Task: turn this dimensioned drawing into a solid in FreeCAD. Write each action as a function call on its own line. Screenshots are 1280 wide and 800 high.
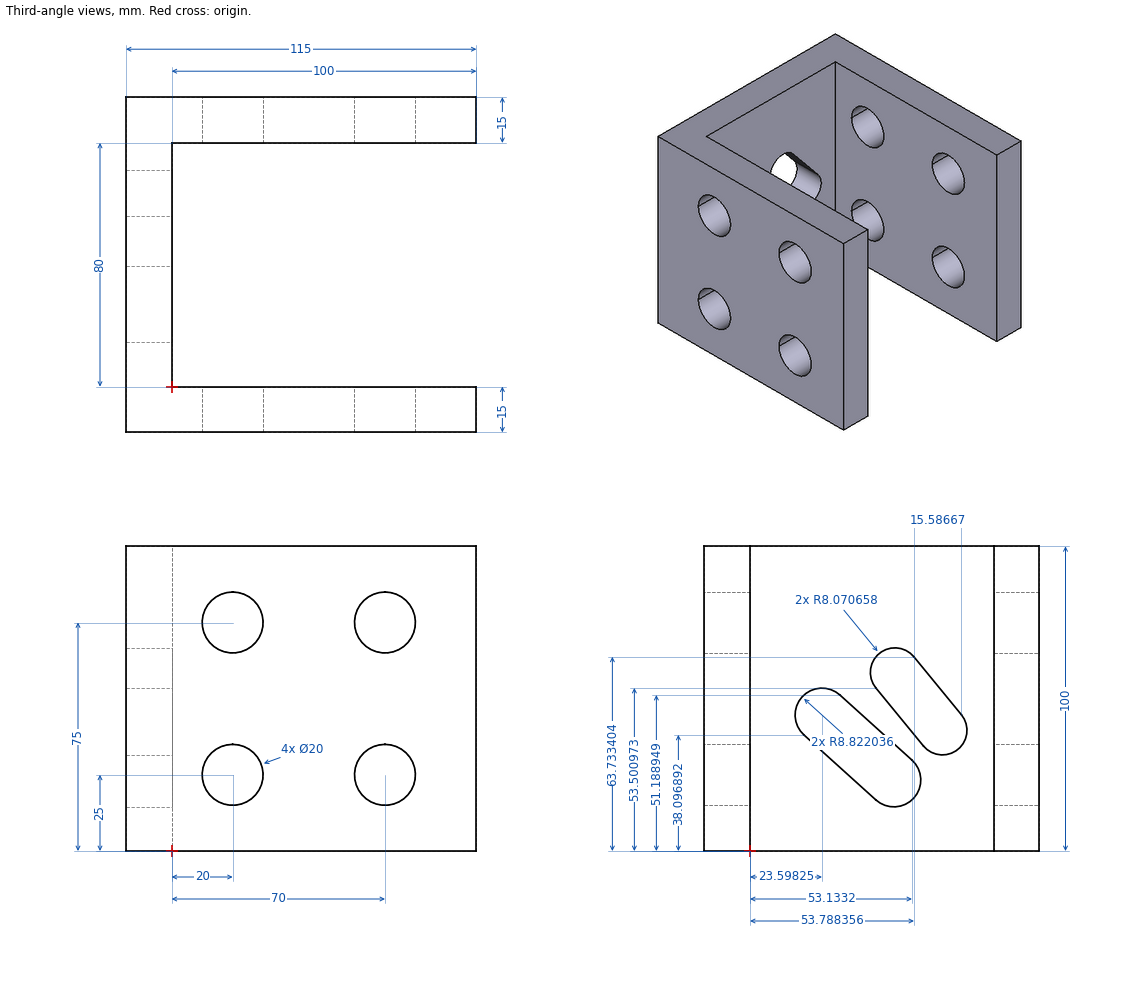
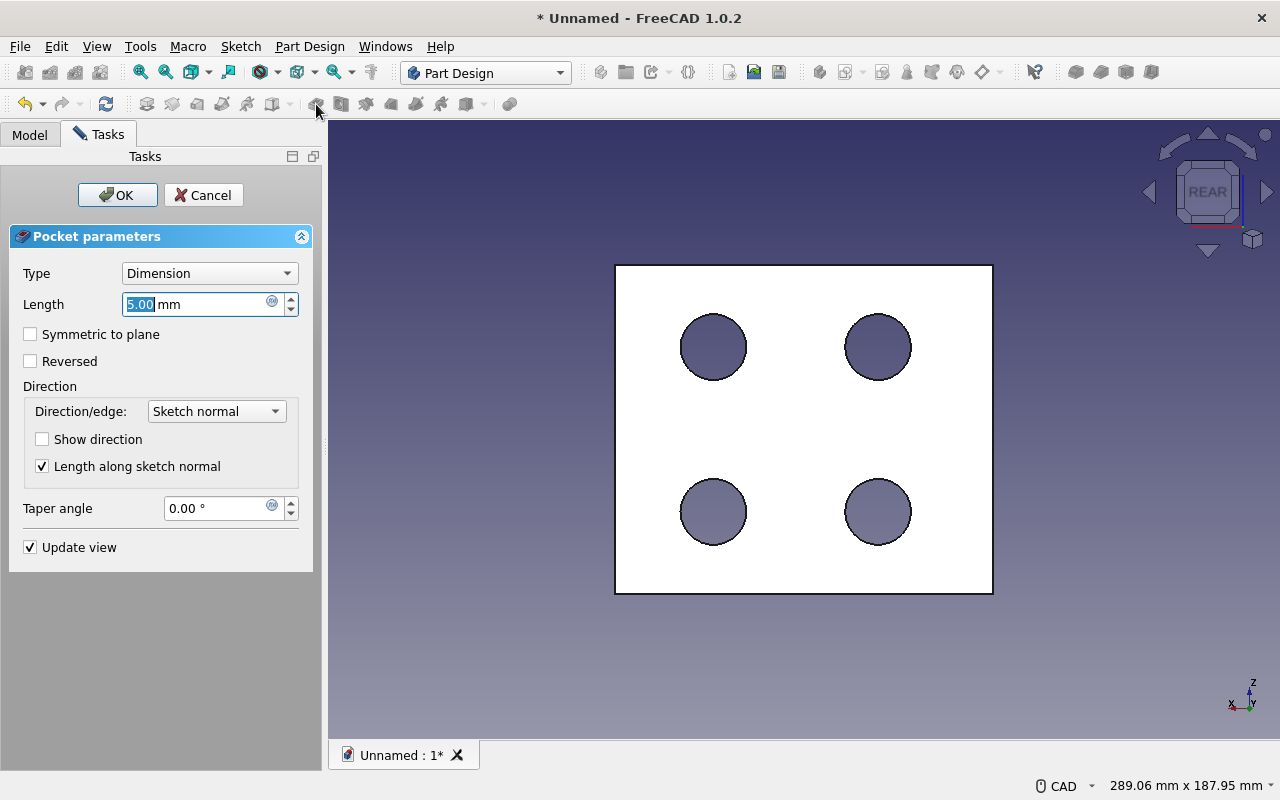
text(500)
key(Tab)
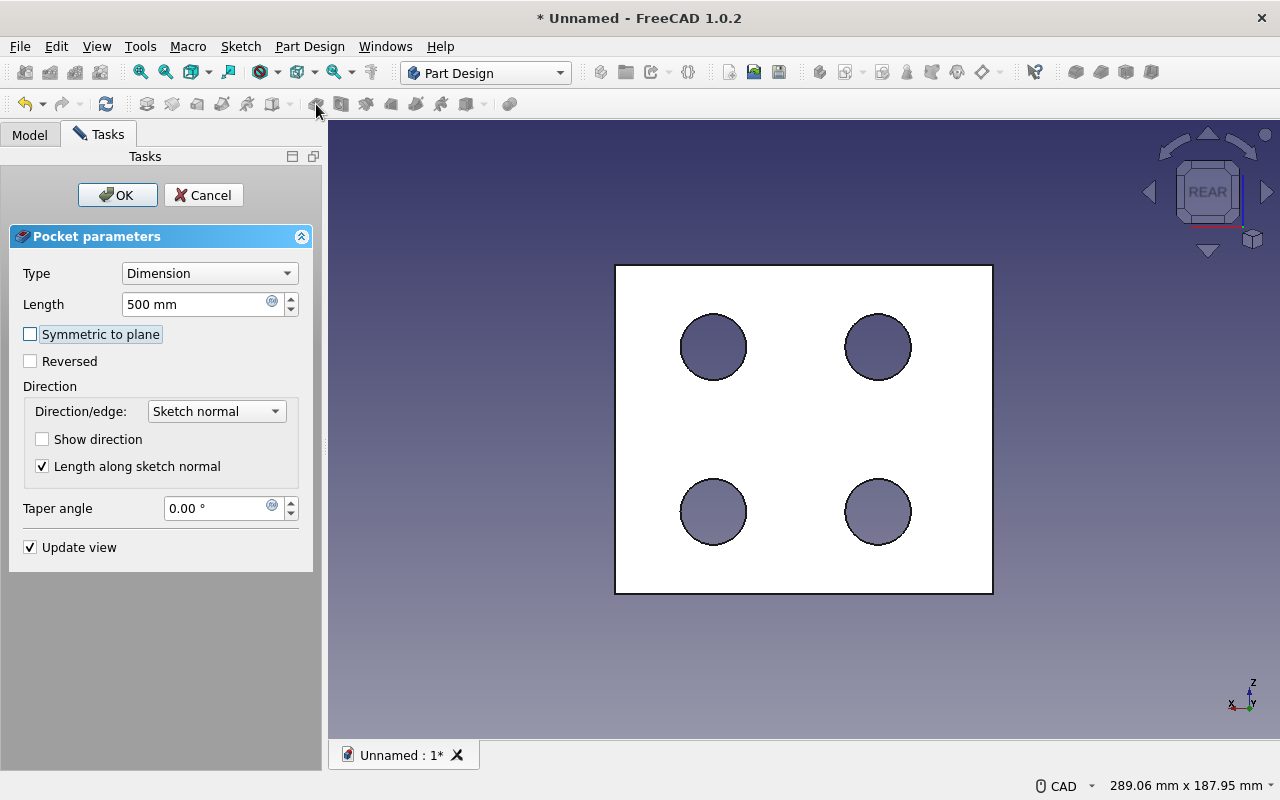
click(118, 195)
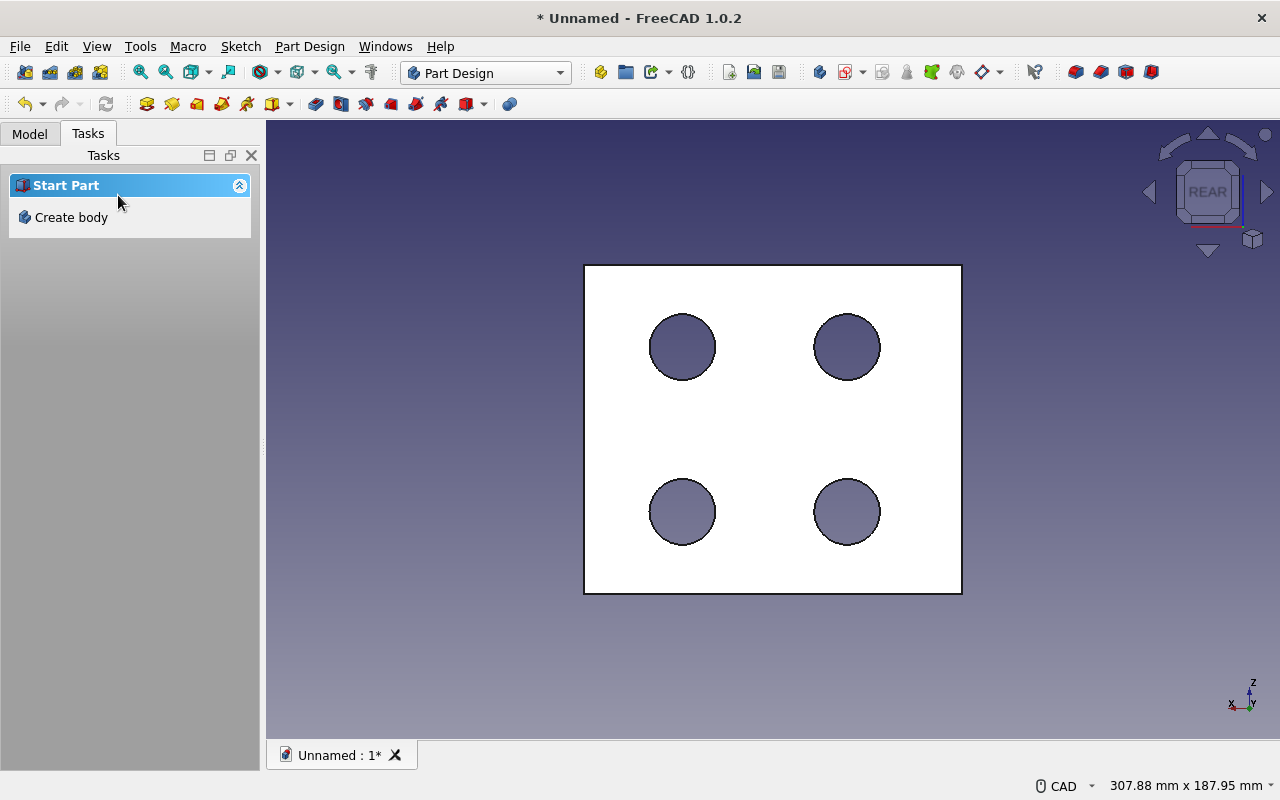
key(0)